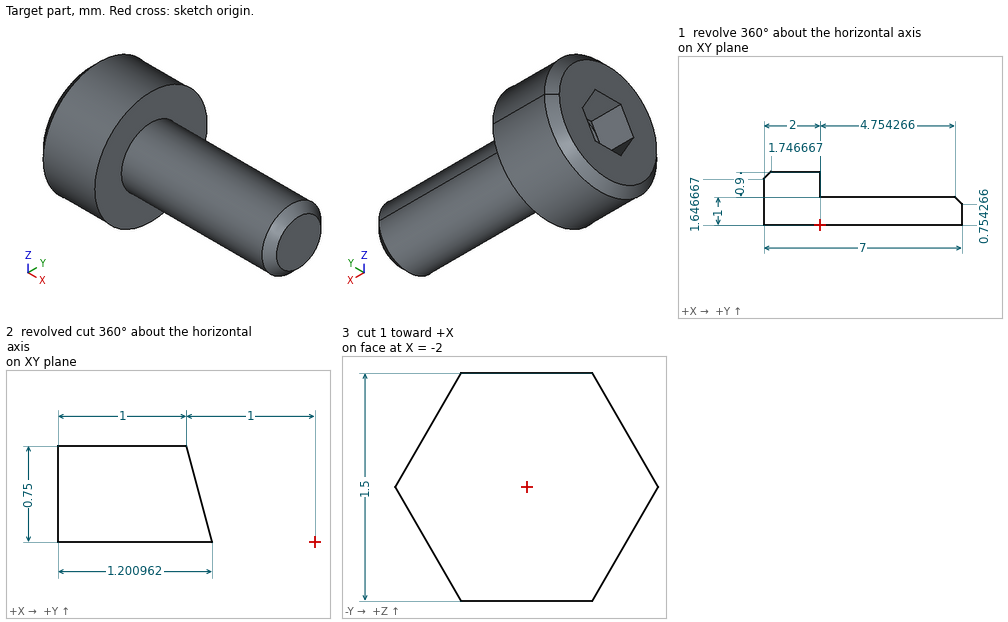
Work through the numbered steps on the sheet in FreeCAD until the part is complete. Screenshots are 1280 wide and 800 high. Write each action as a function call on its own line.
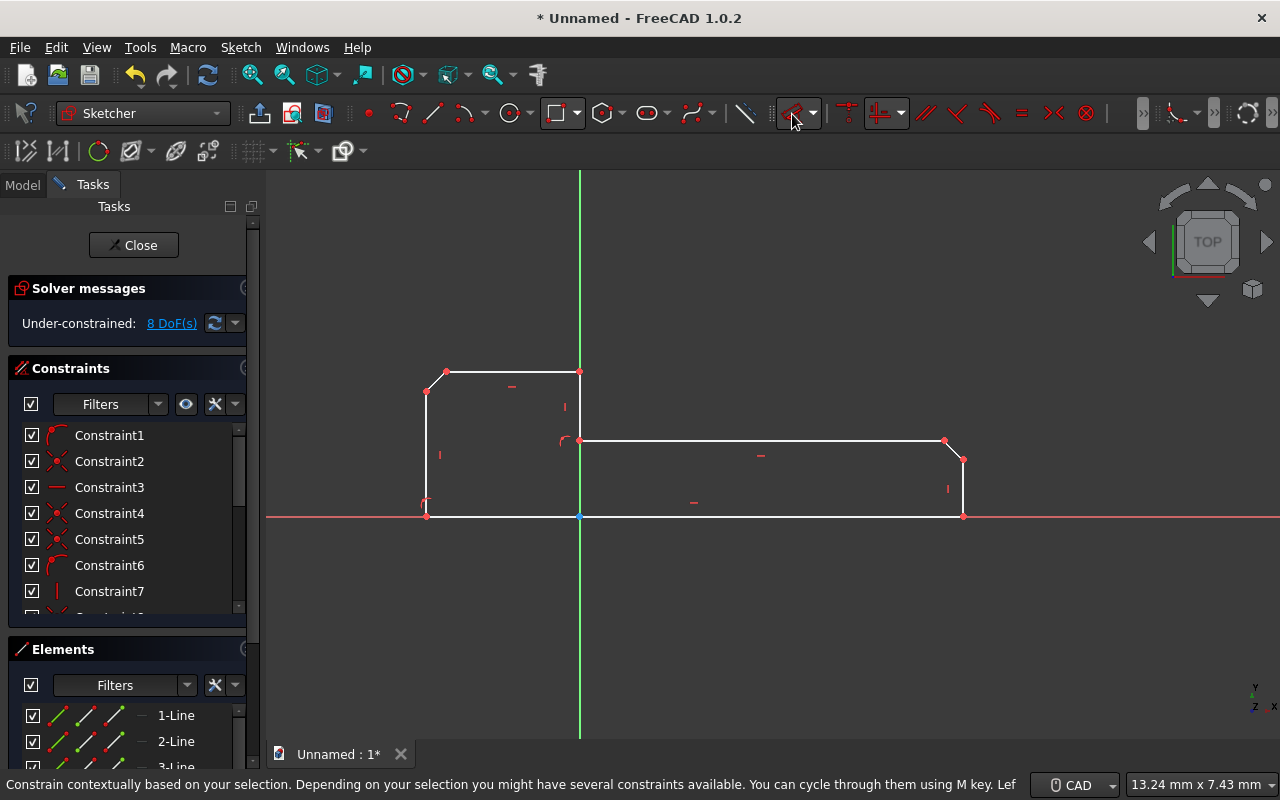
click(802, 517)
click(694, 551)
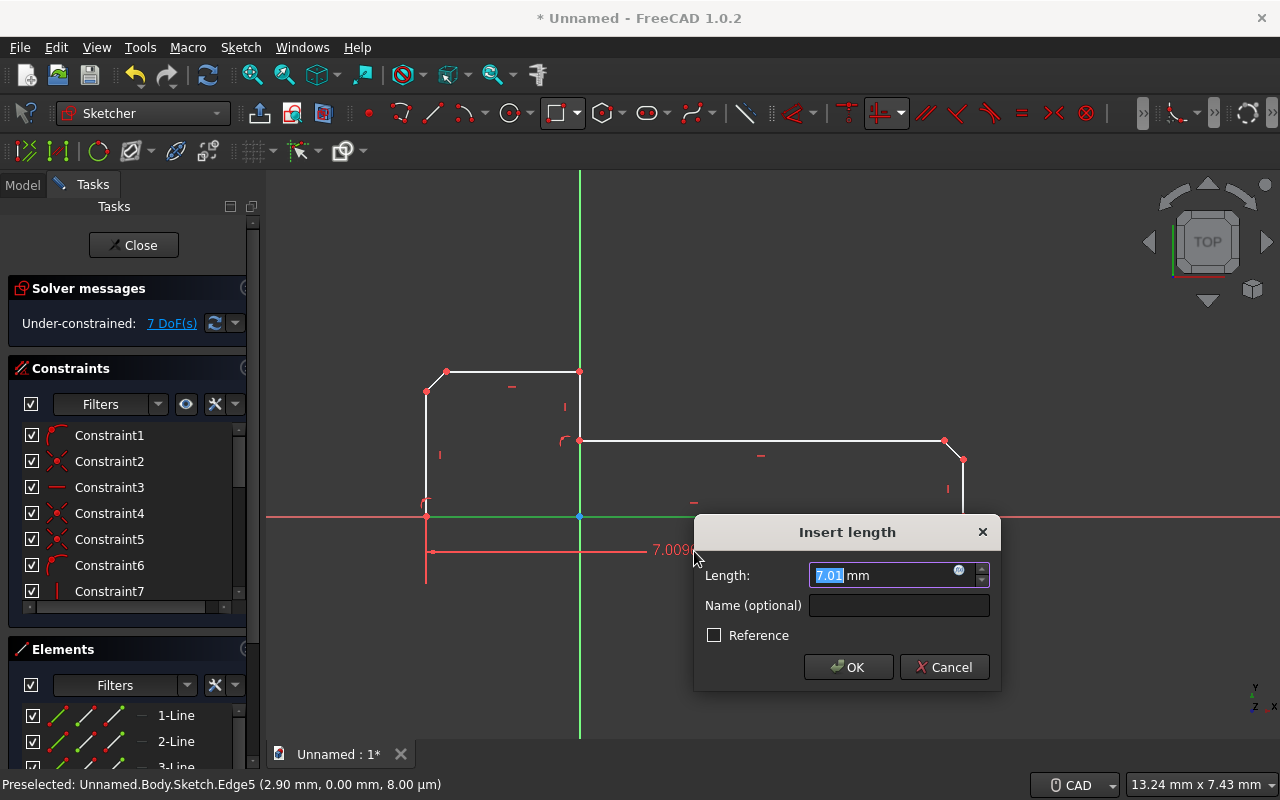
text(7)
key(Return)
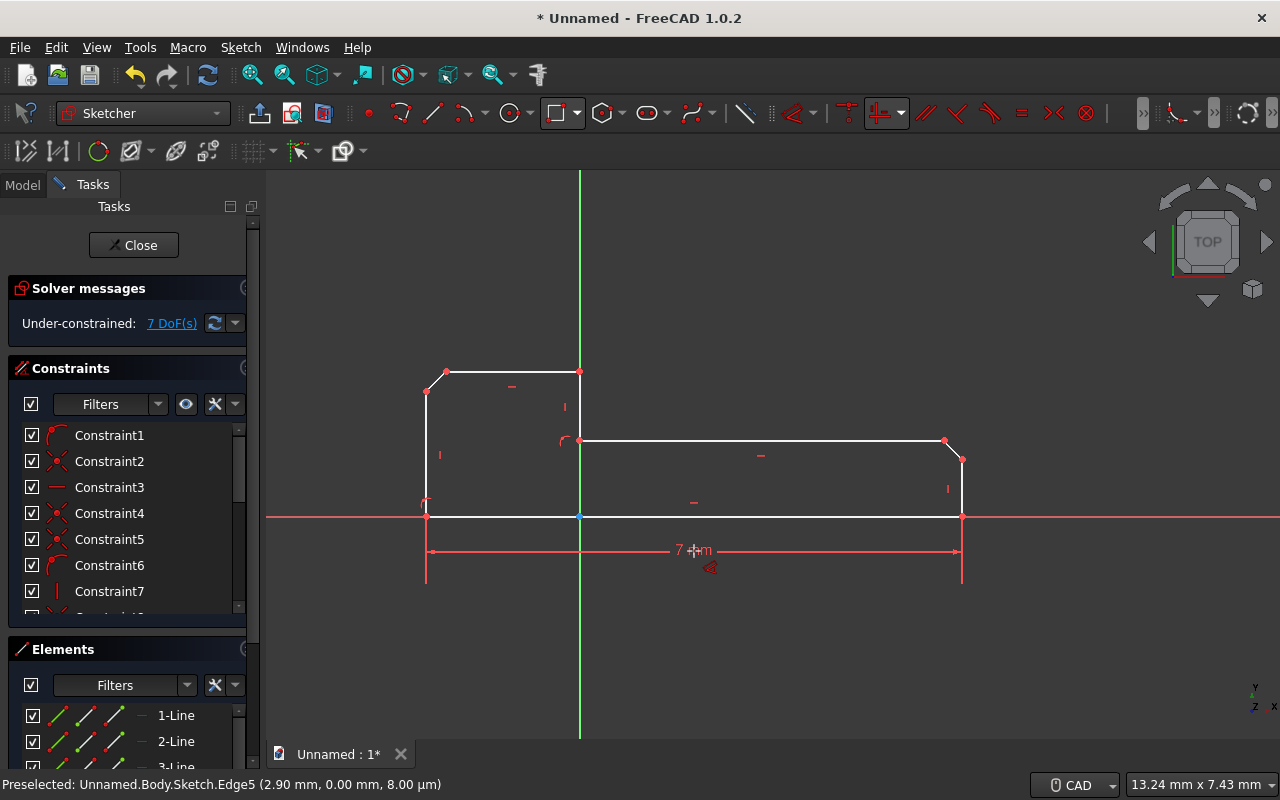
click(580, 441)
click(546, 479)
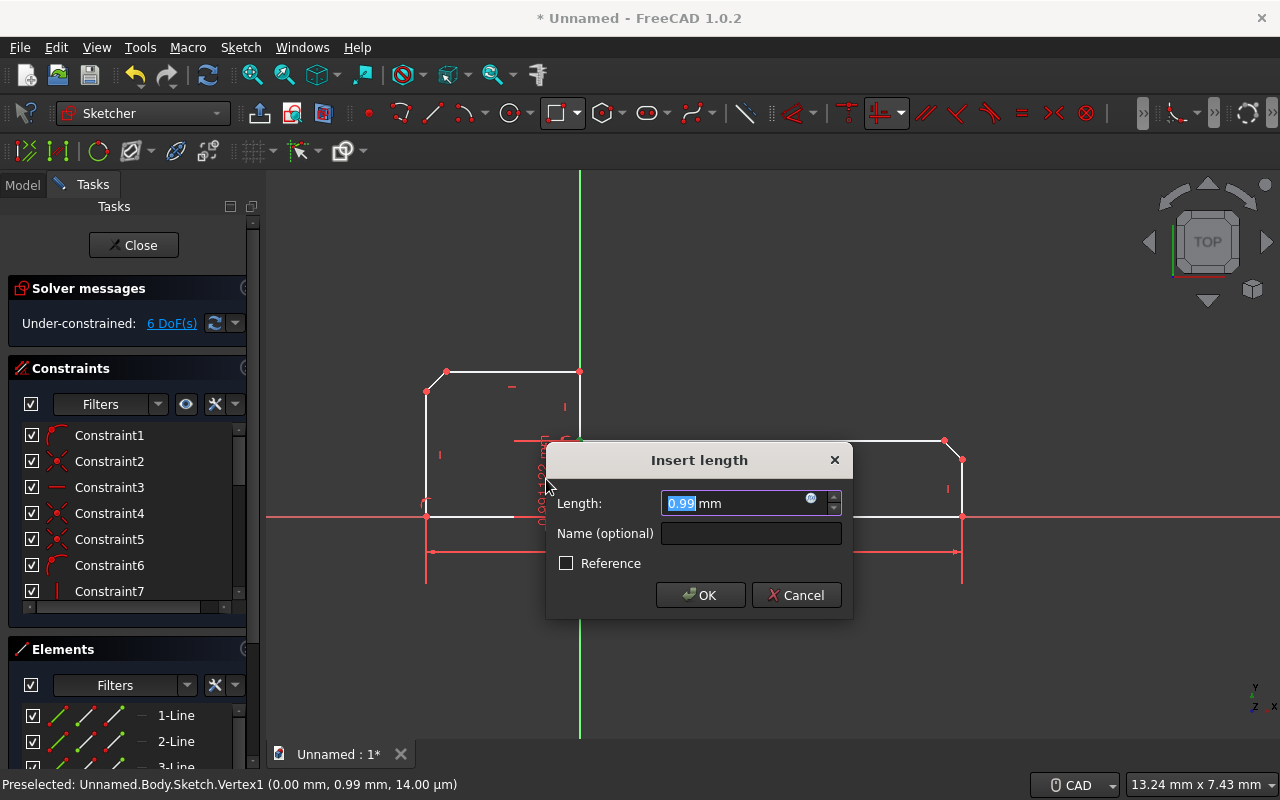
text(1)
key(Return)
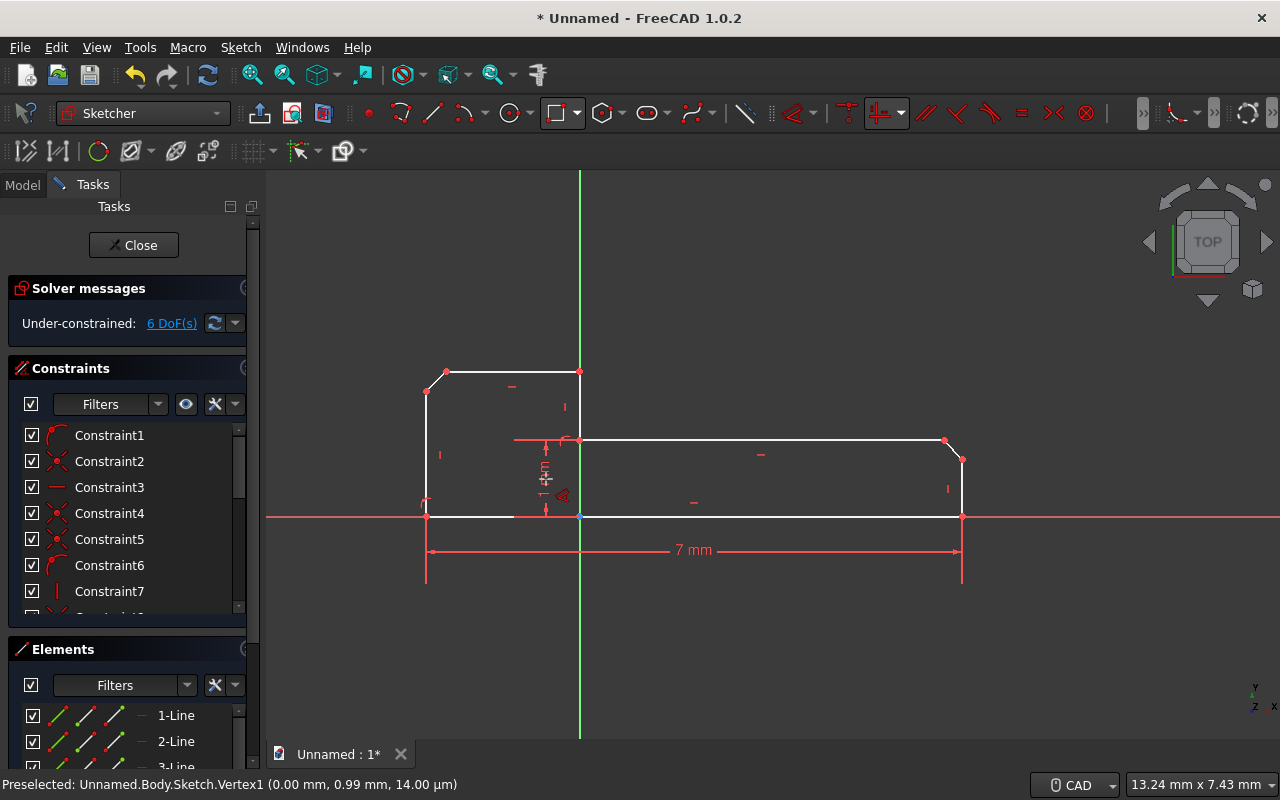
click(426, 392)
click(503, 551)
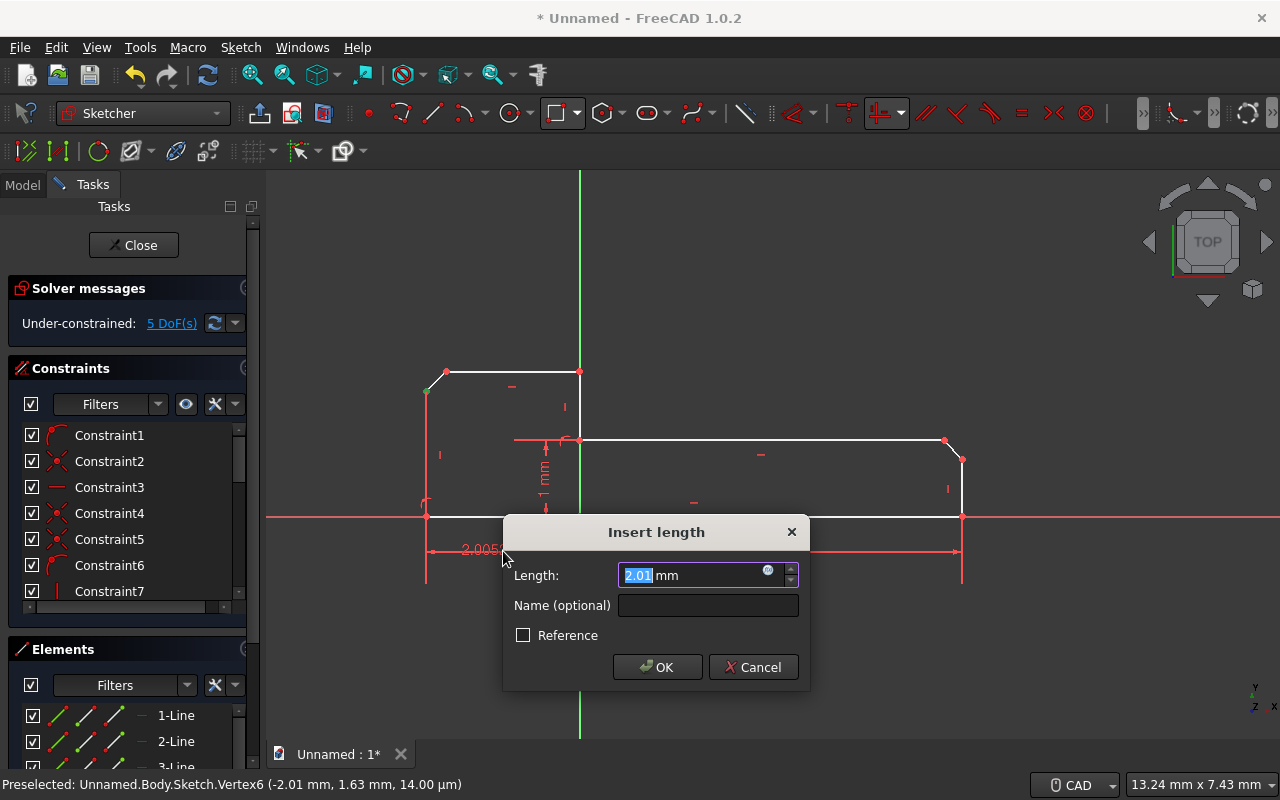
text(2)
key(Return)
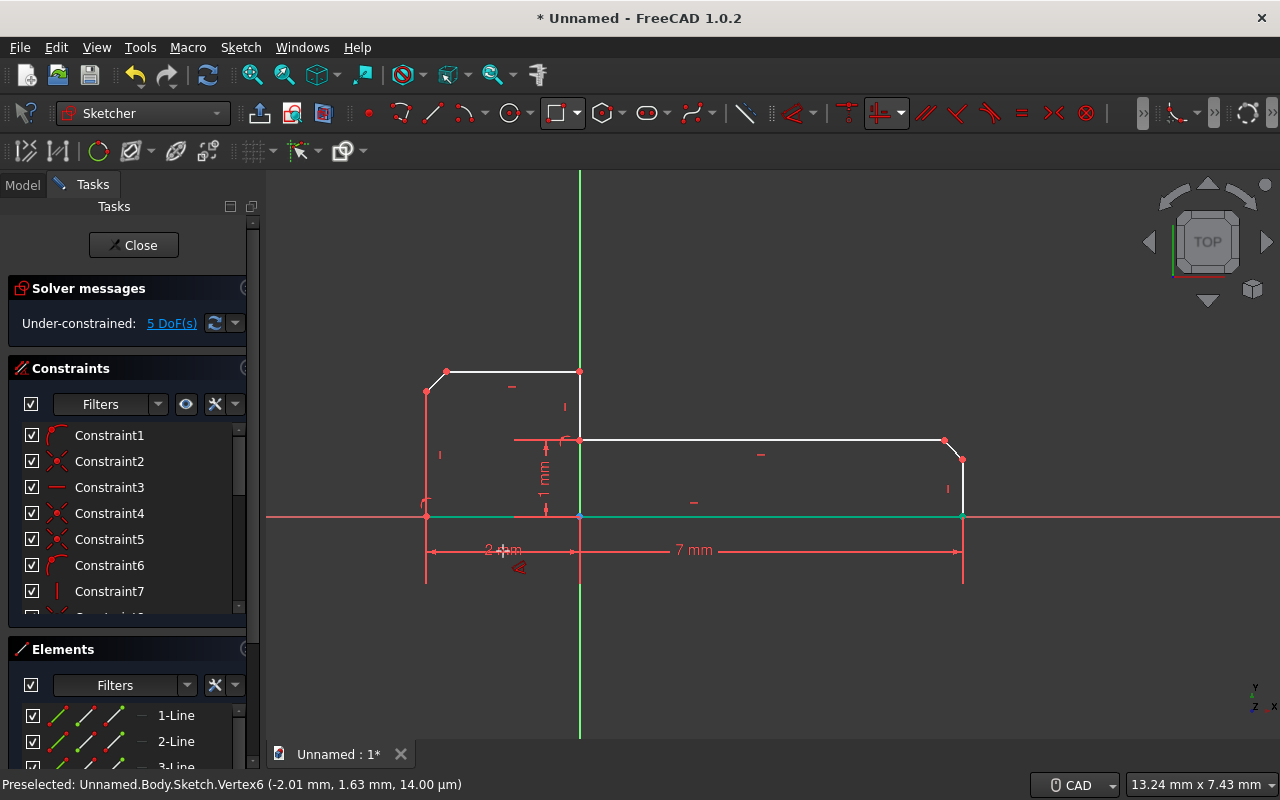
click(580, 420)
click(546, 406)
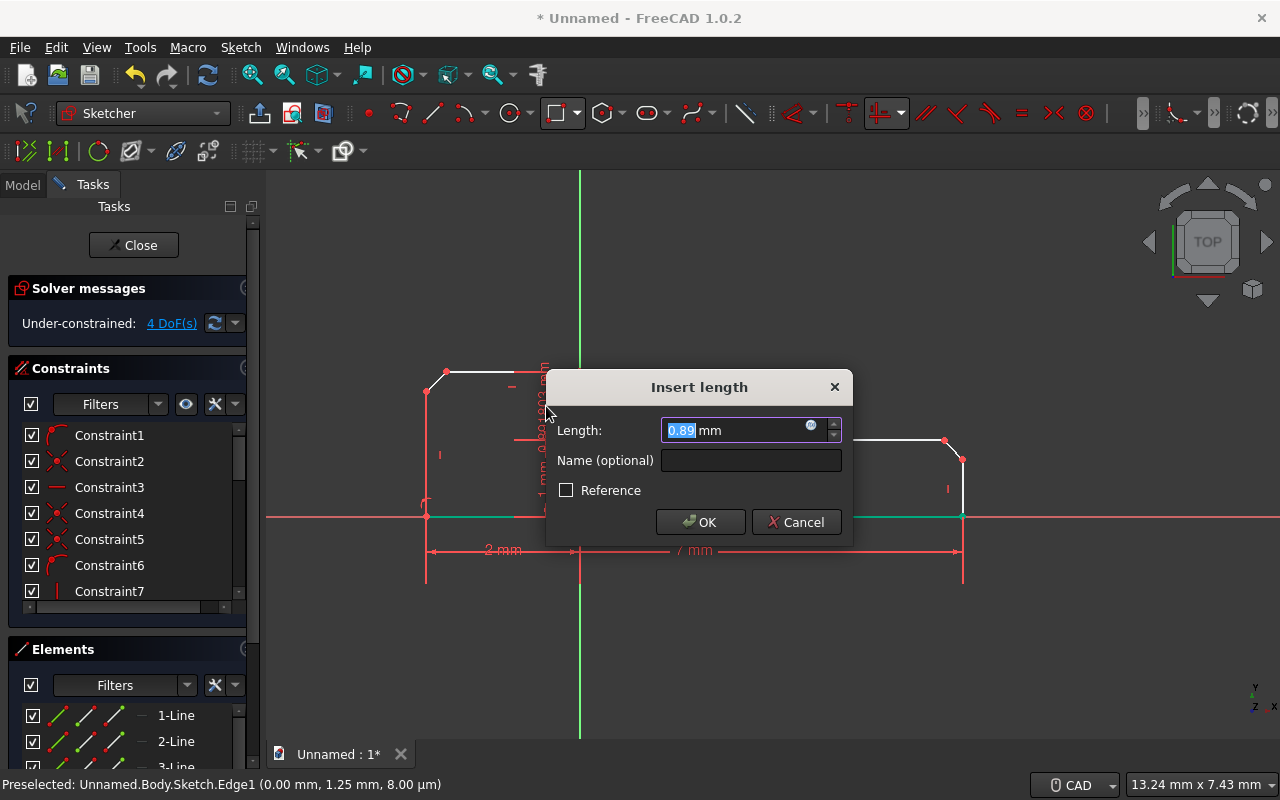
text(0.9)
key(Return)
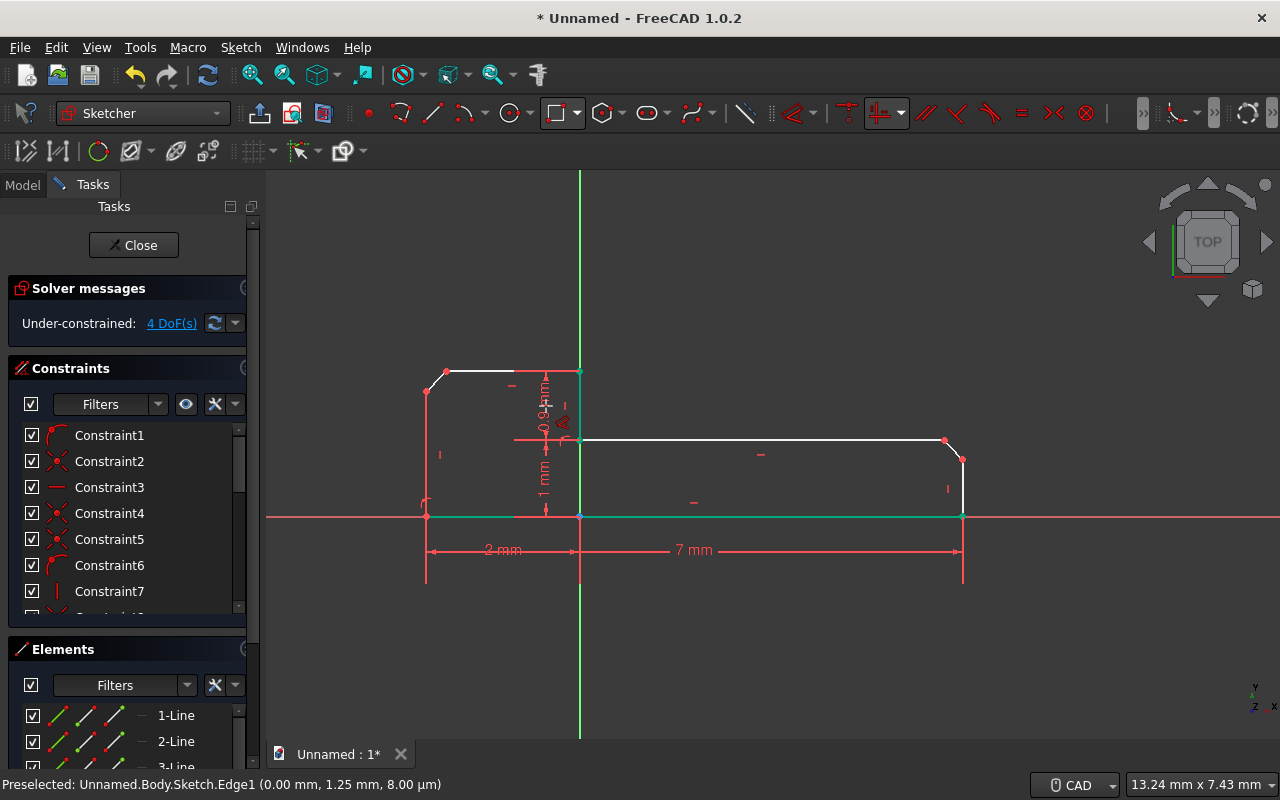
click(540, 371)
click(513, 337)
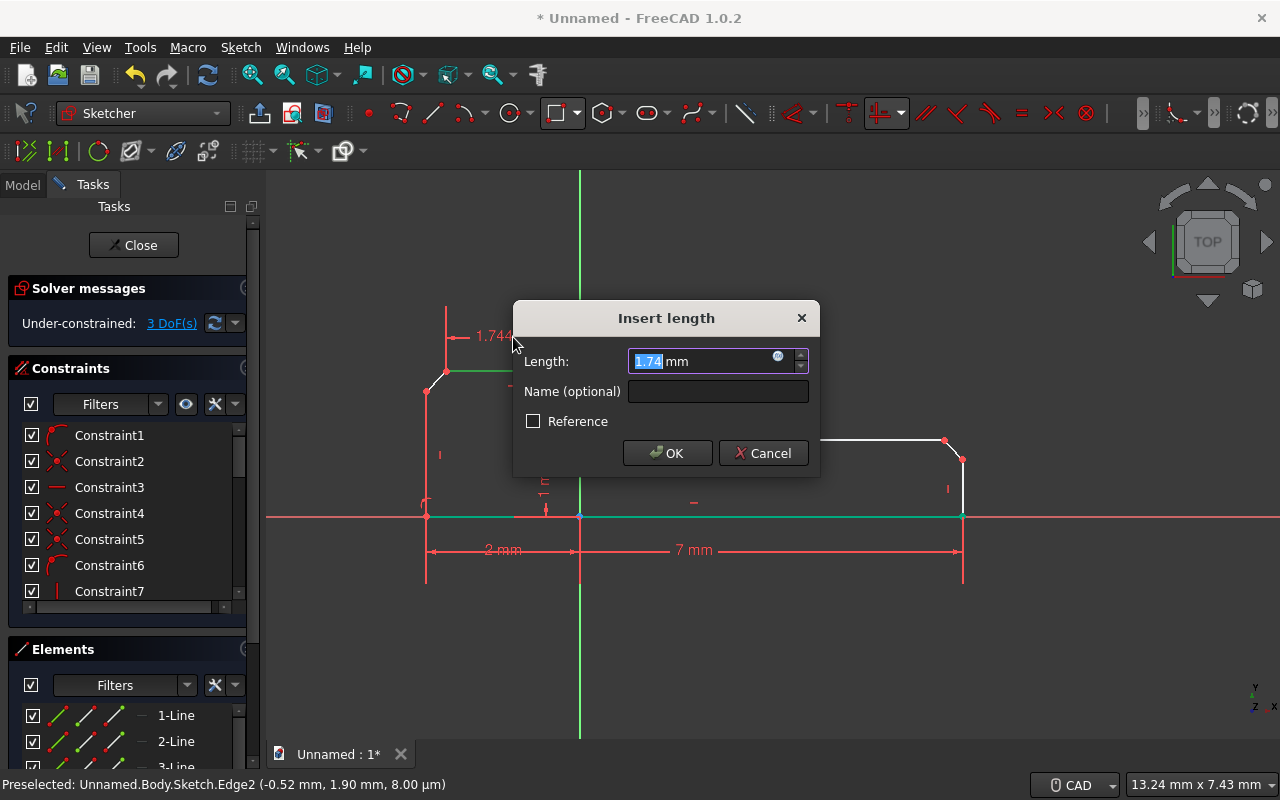
text(1.746667)
key(Return)